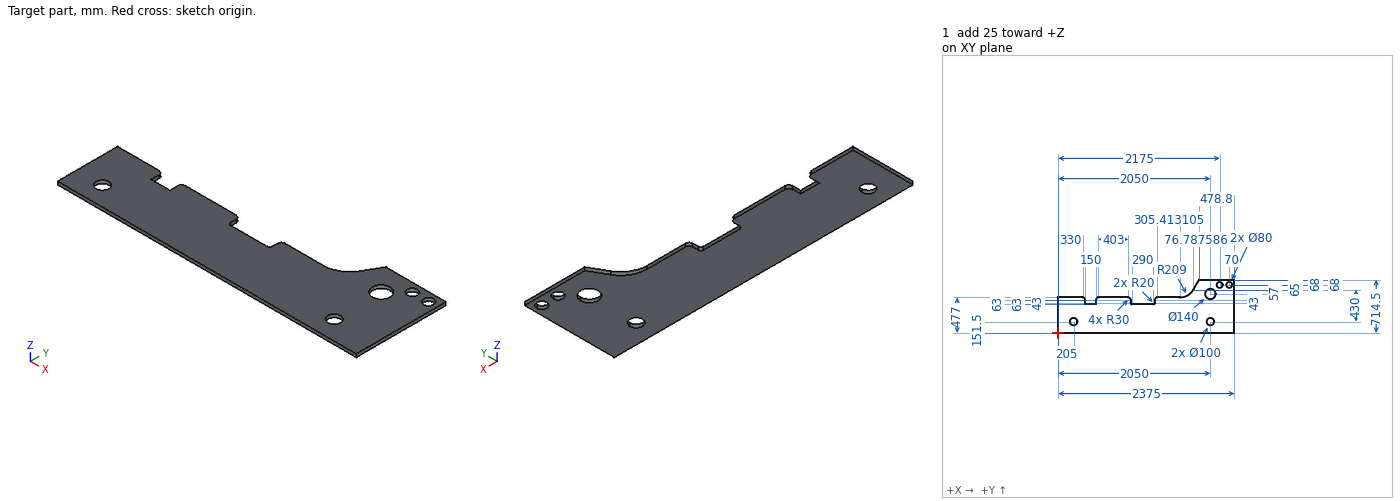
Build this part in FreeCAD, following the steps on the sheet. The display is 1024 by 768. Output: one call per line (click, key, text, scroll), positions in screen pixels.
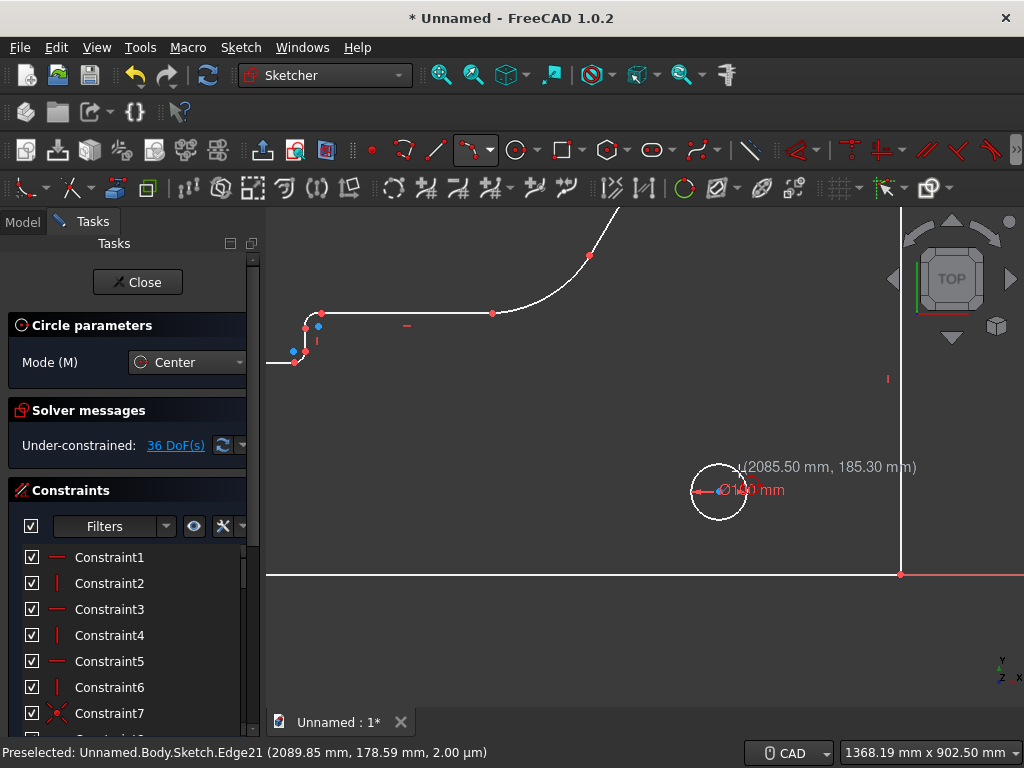
scroll(721, 492, down, 6)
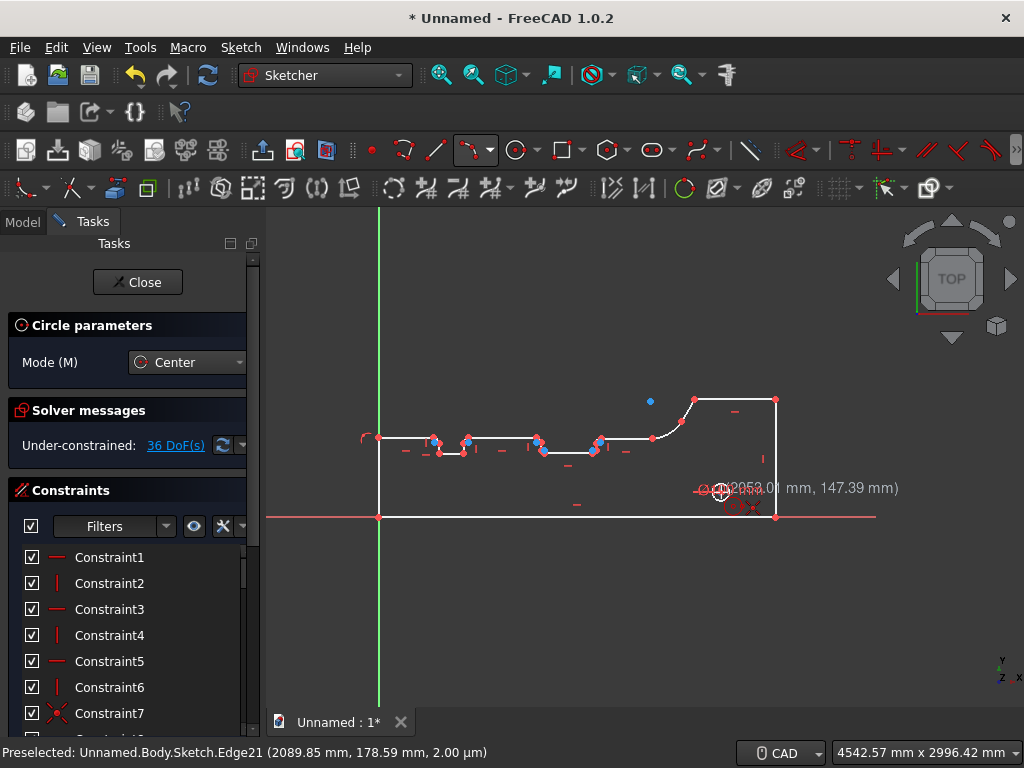
scroll(413, 492, up, 6)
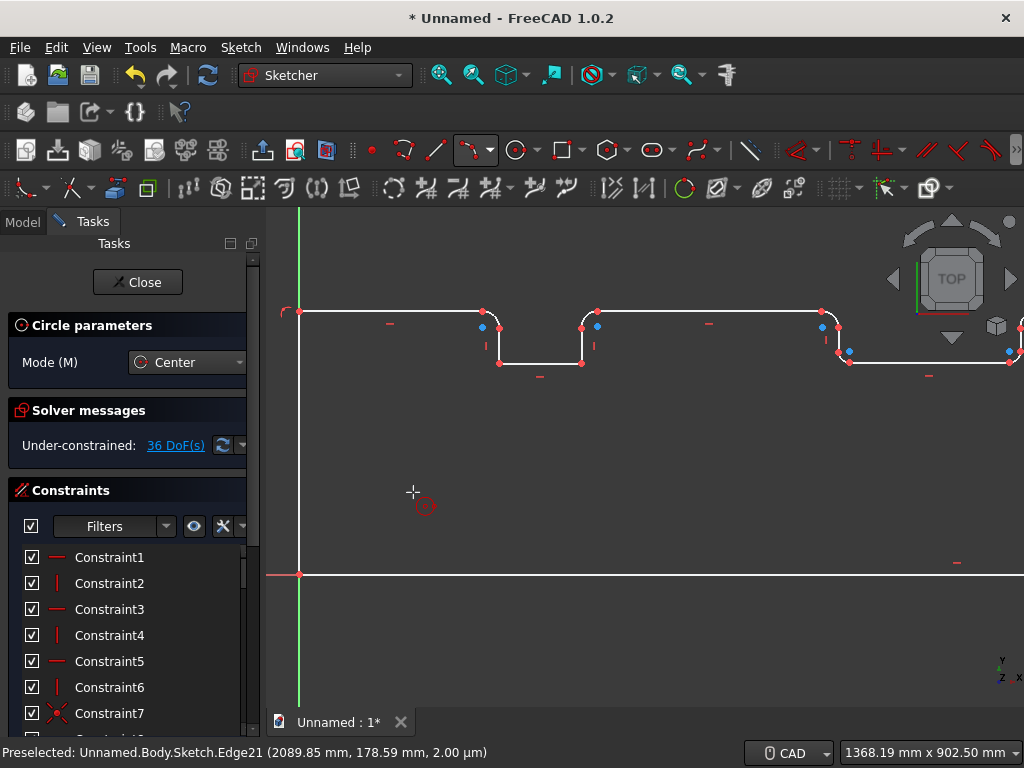
click(413, 491)
move(432, 471)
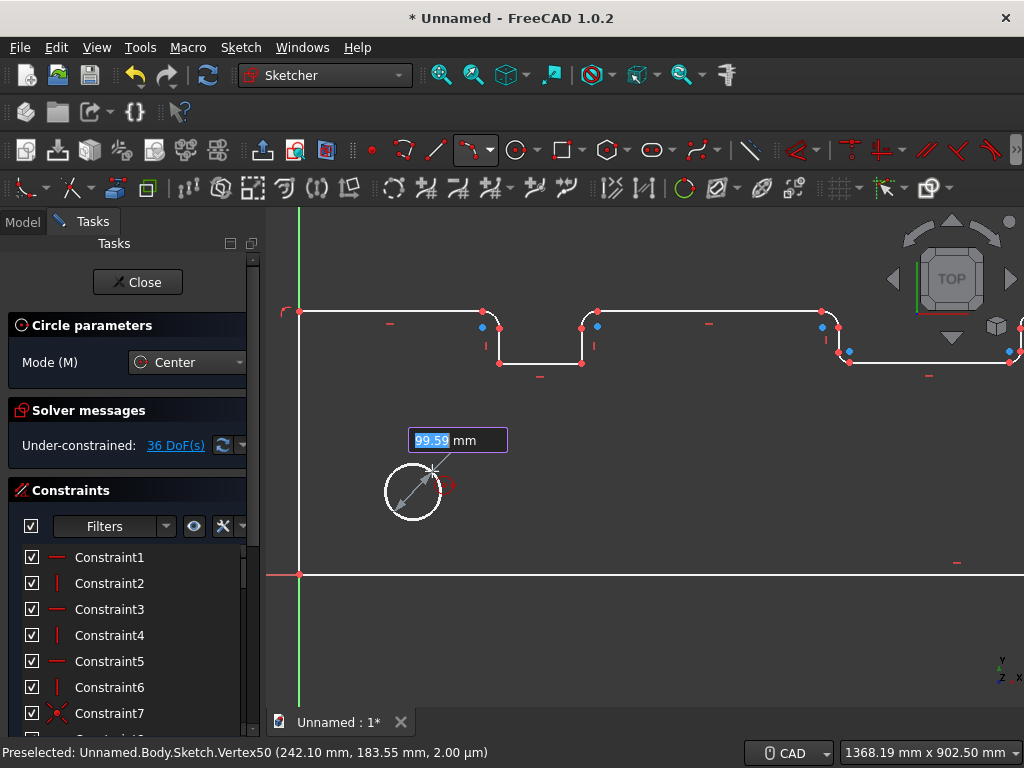
text(100)
key(Return)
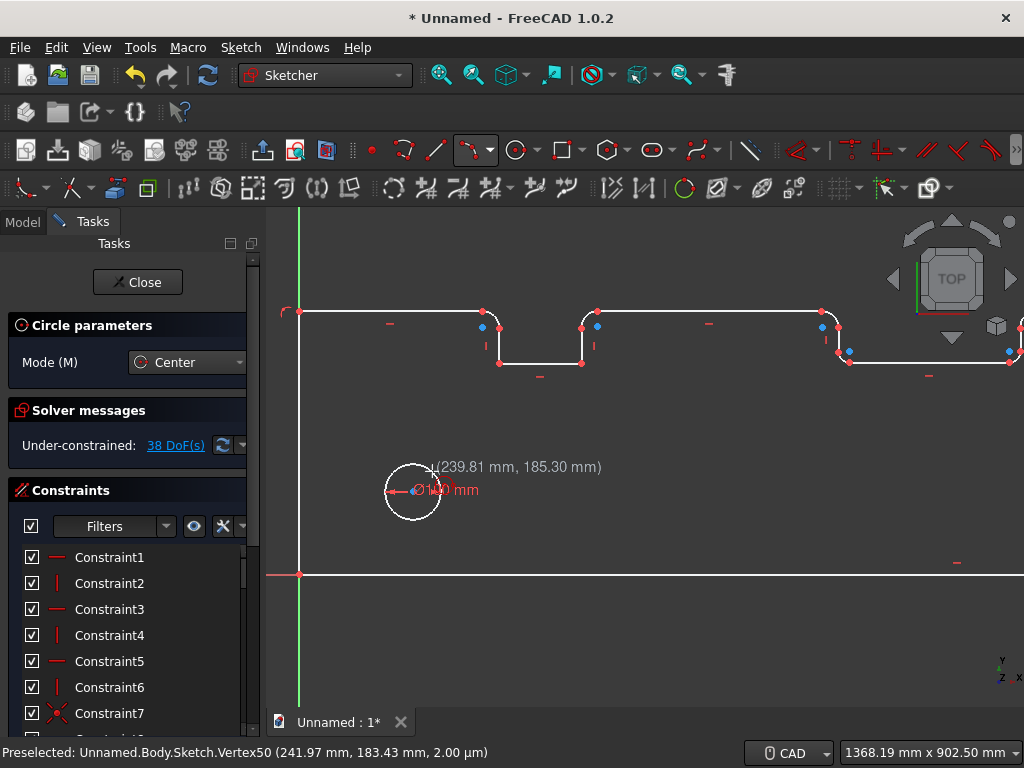
scroll(412, 492, down, 6)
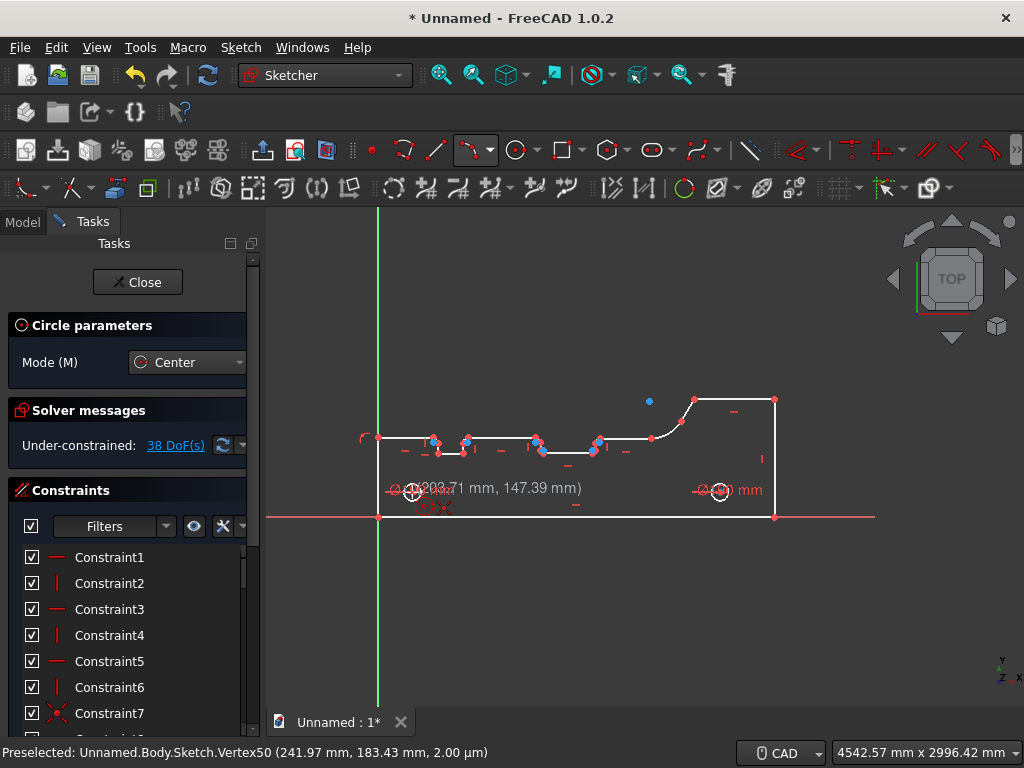
scroll(720, 430, up, 4)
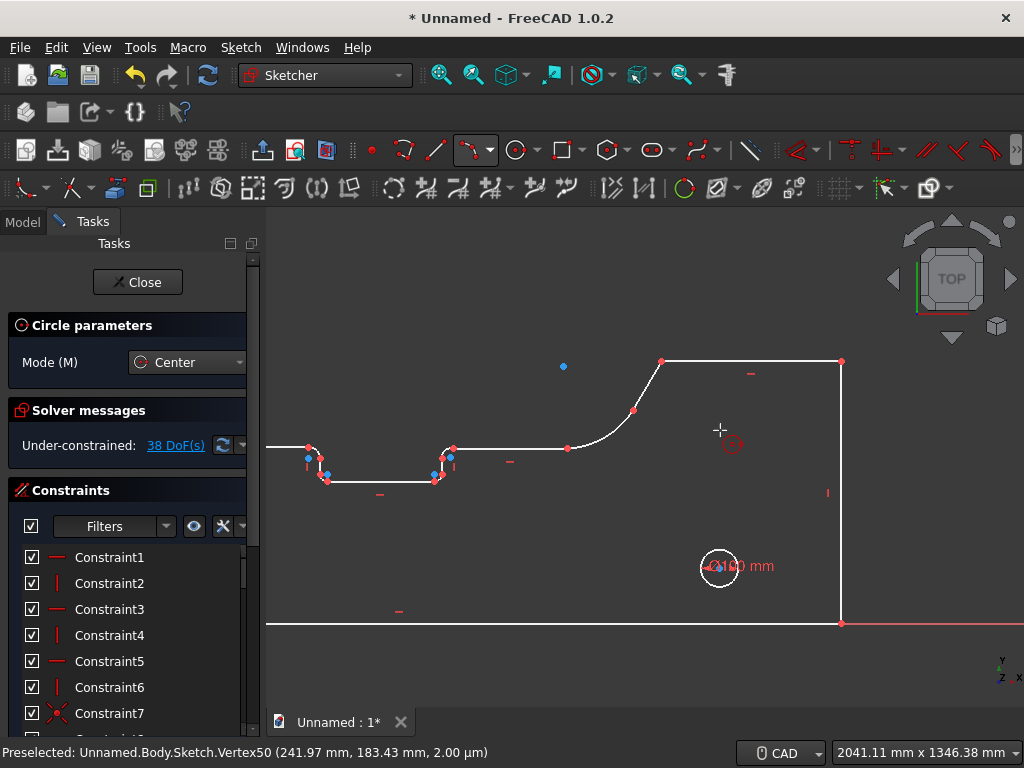
click(720, 429)
move(738, 411)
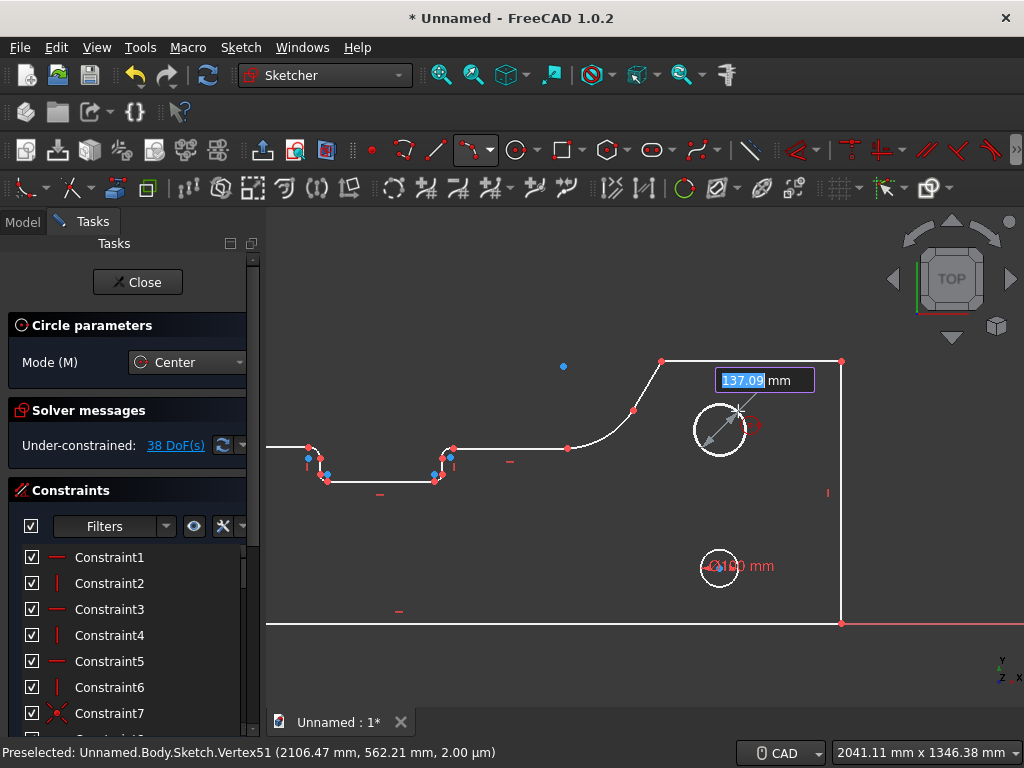
text(140)
key(Return)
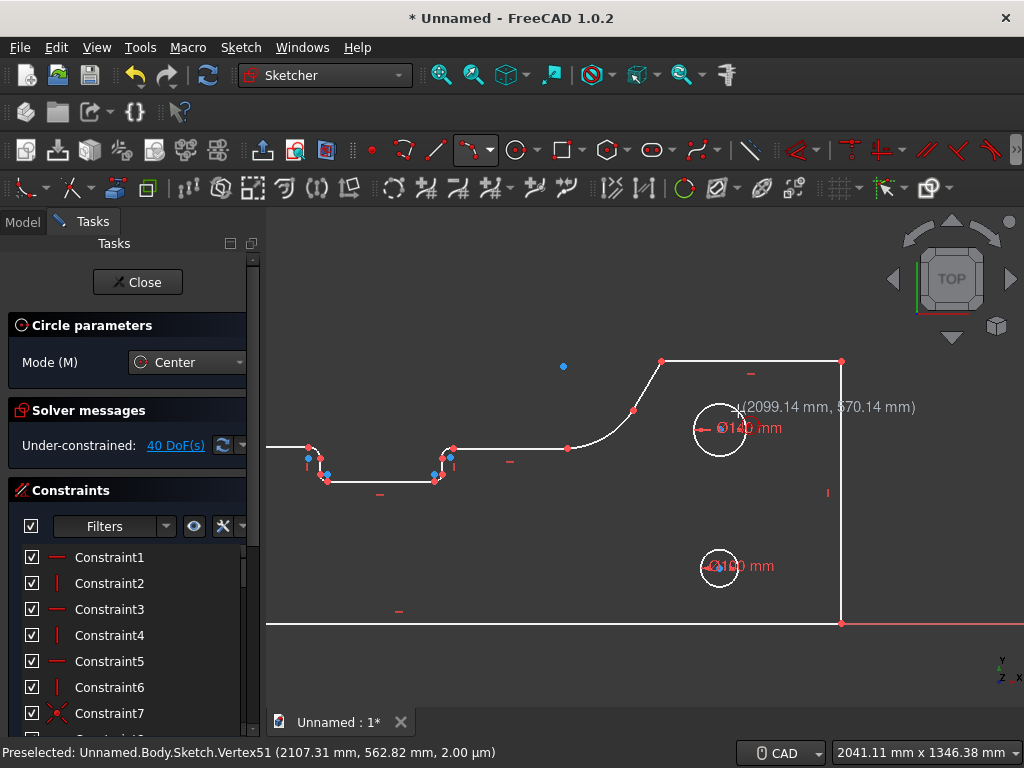
scroll(814, 384, up, 3)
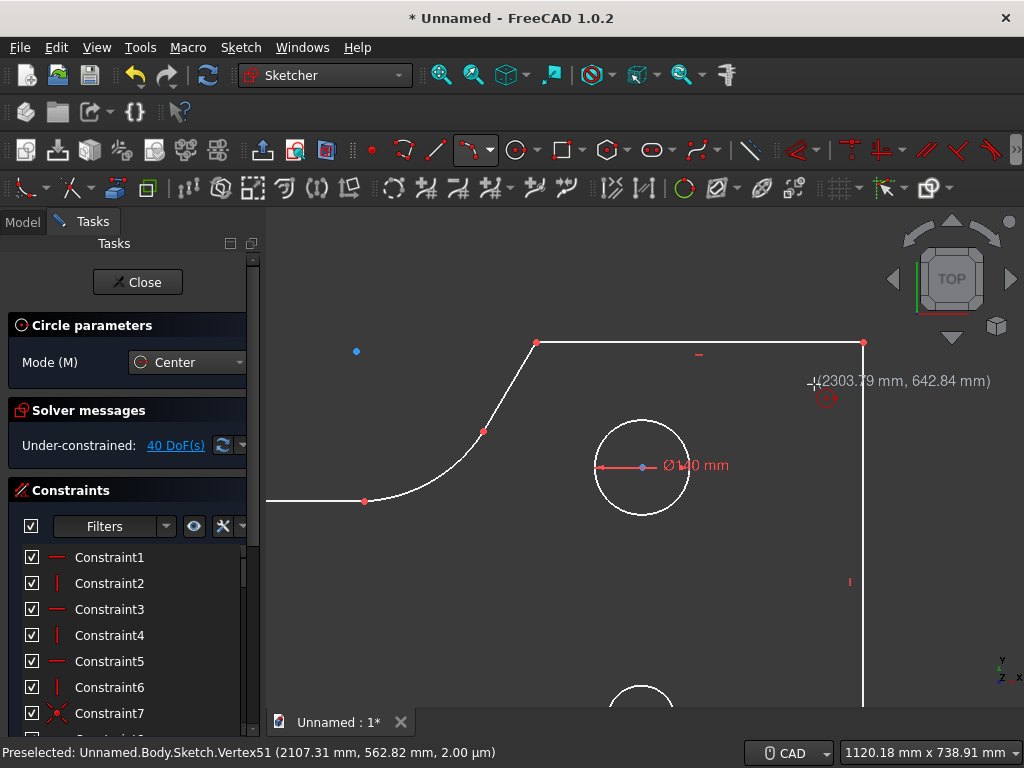
click(814, 383)
move(833, 364)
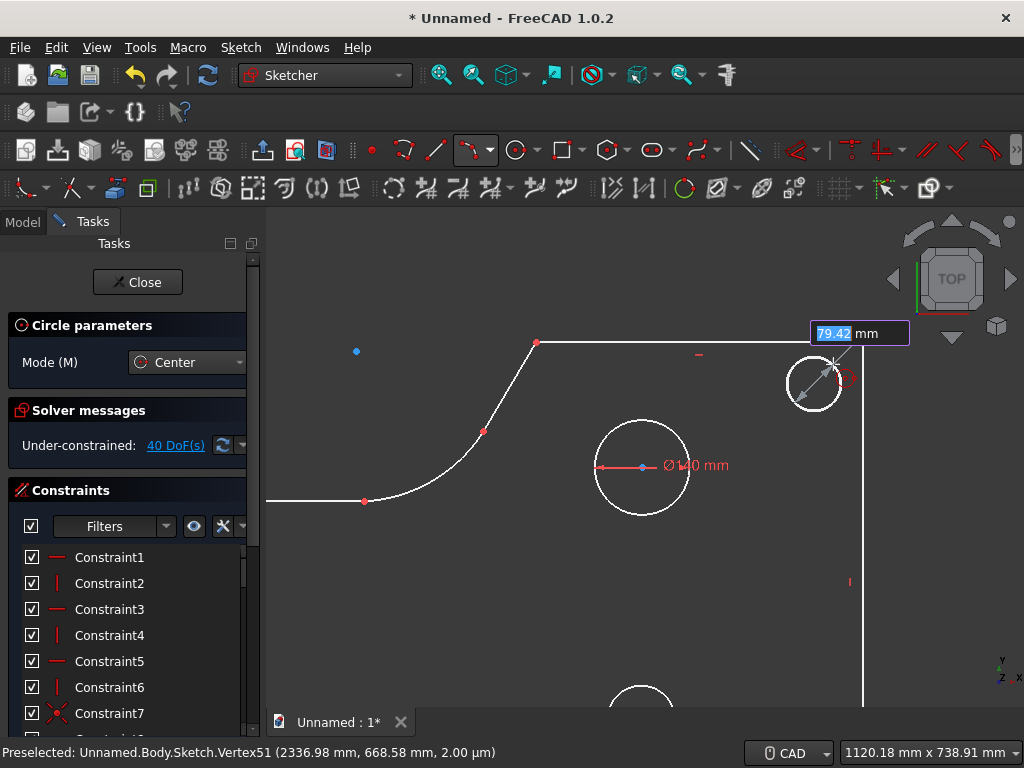
text(80)
key(Return)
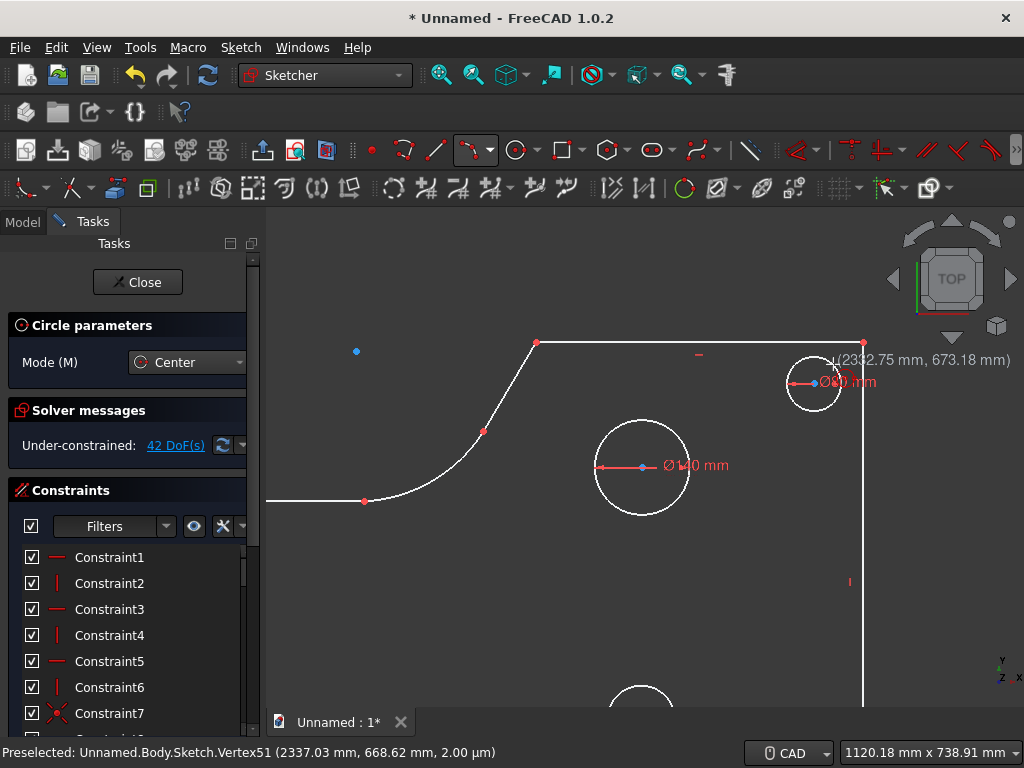
click(726, 383)
move(745, 364)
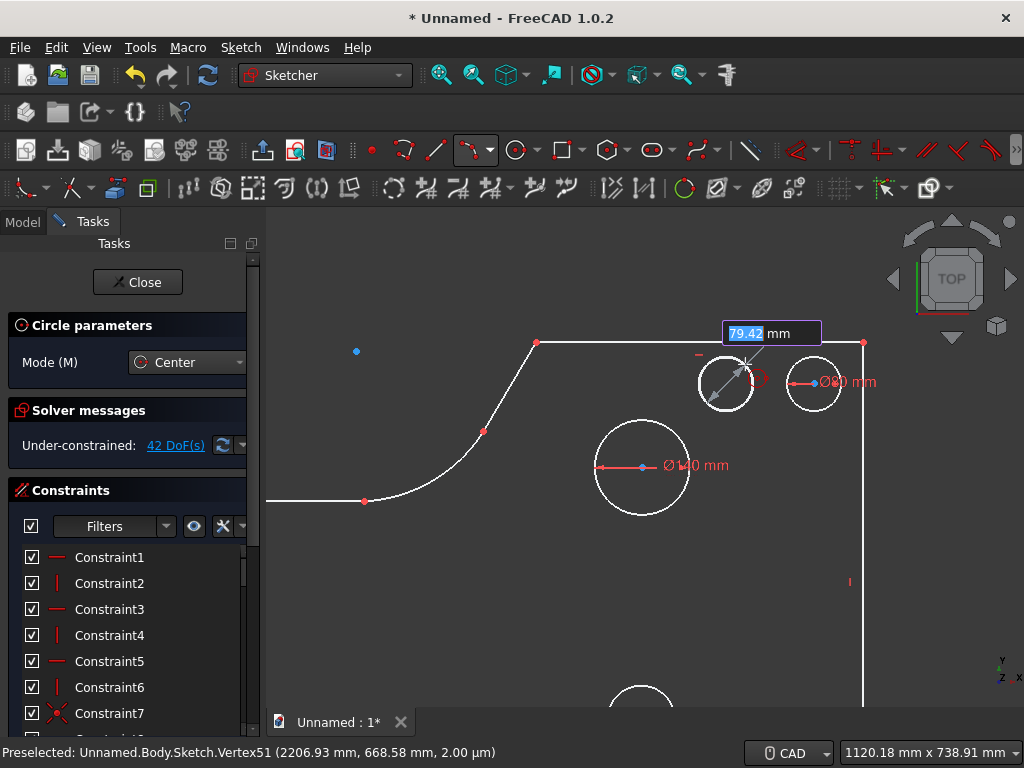
text(80)
key(Return)
key(Escape)